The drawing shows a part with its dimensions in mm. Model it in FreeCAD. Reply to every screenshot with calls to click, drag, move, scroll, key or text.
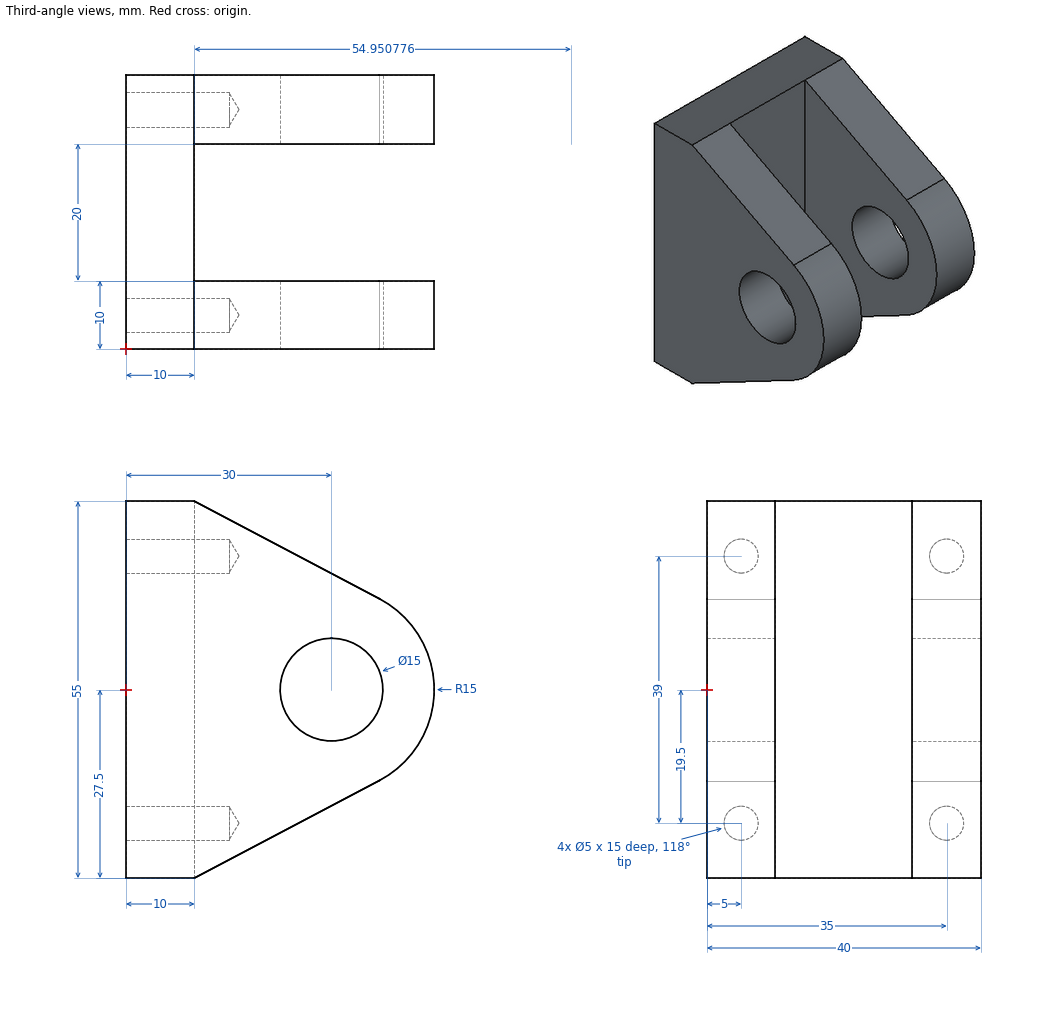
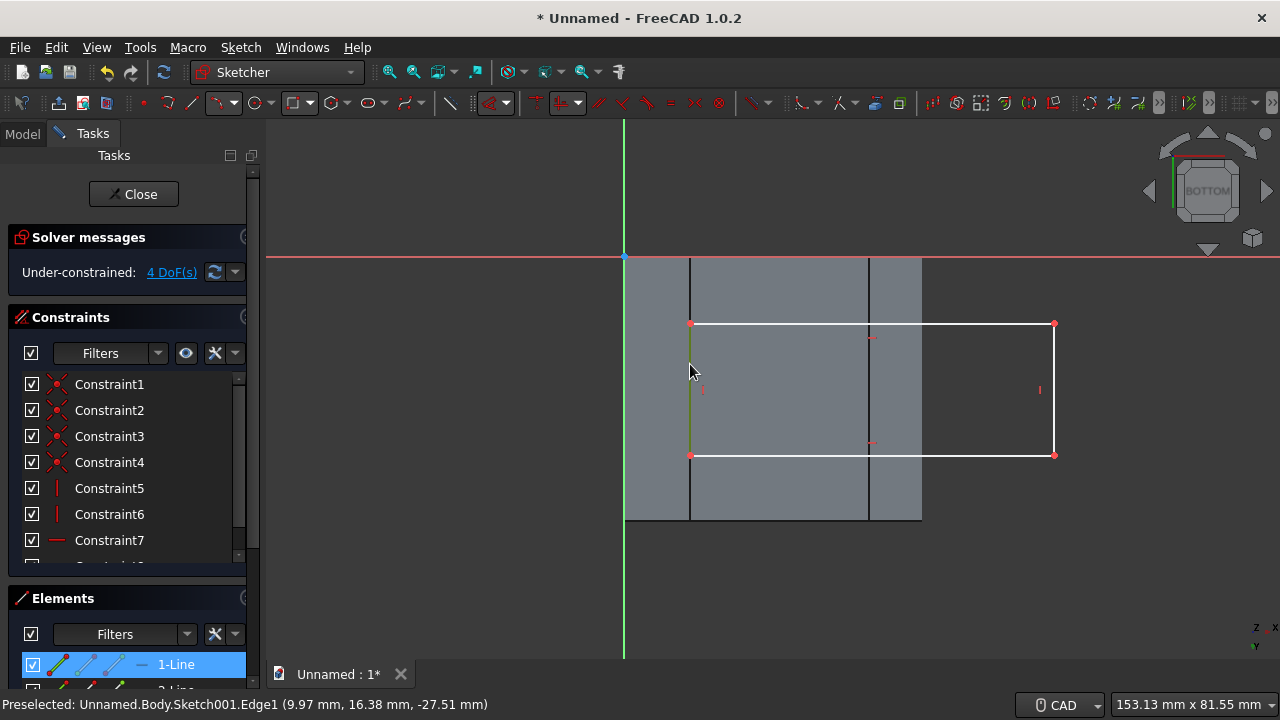
key(i)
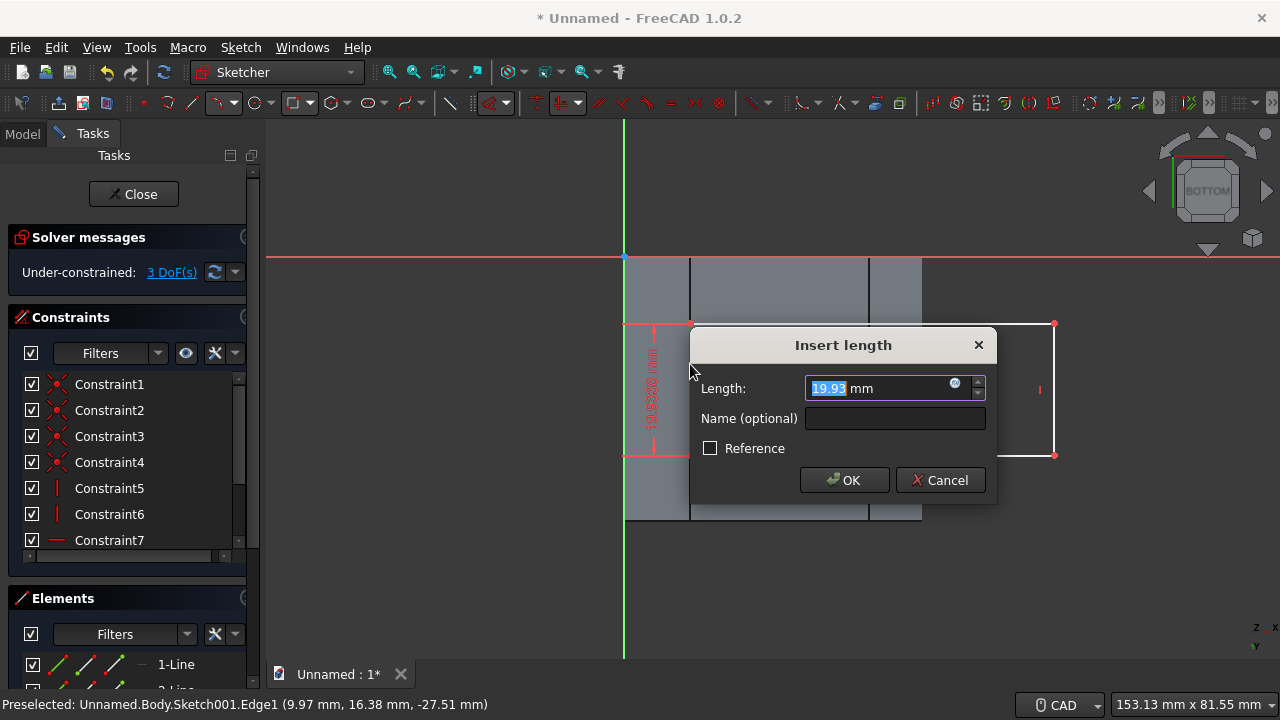
text(20)
key(Return)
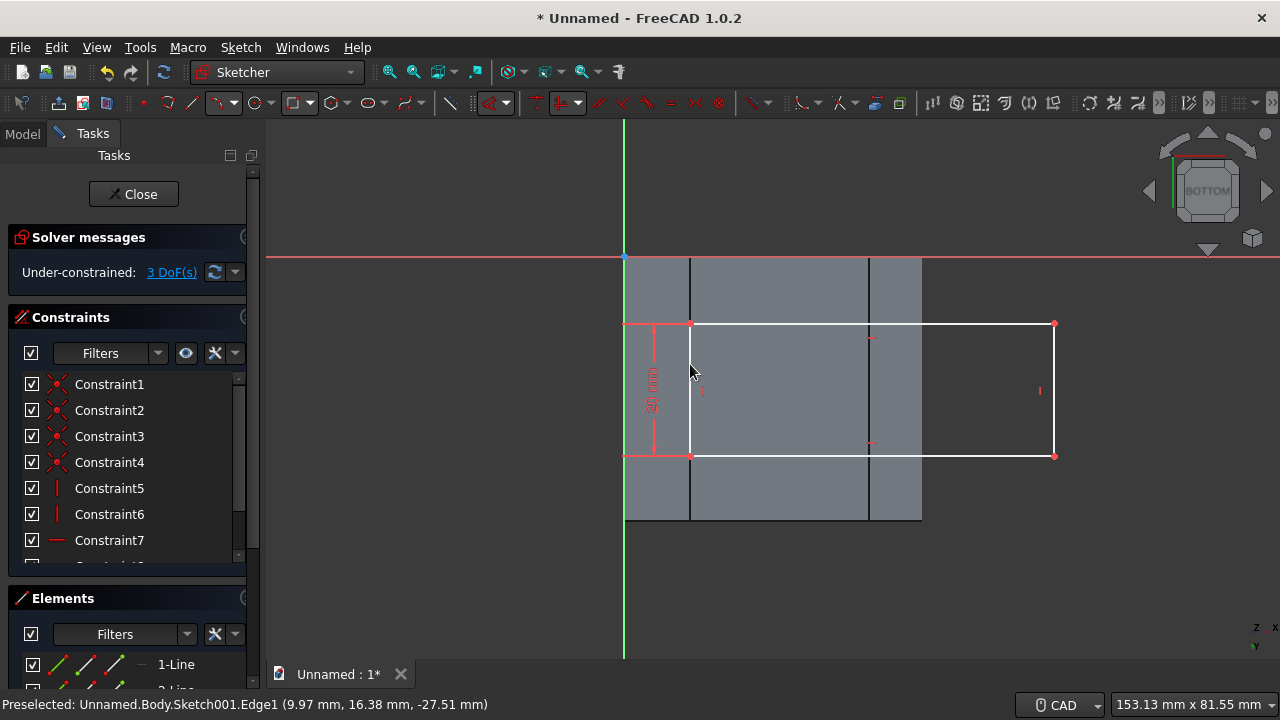
click(690, 324)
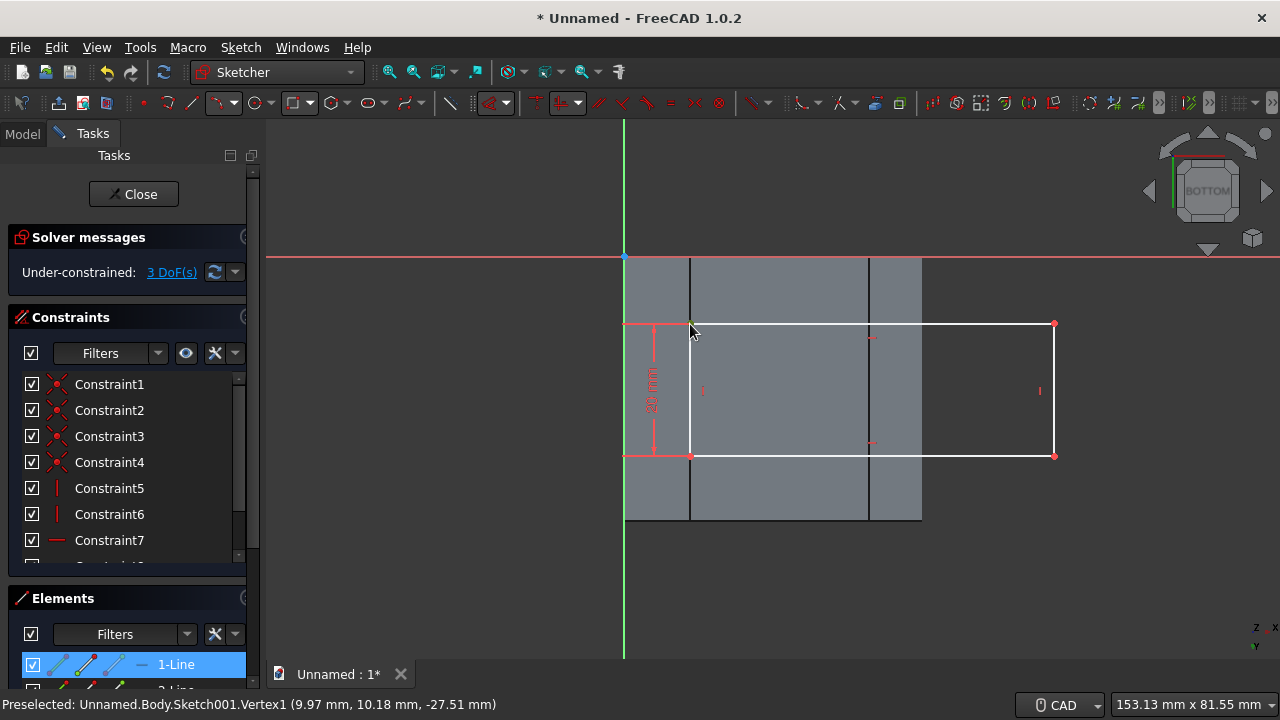
key(l)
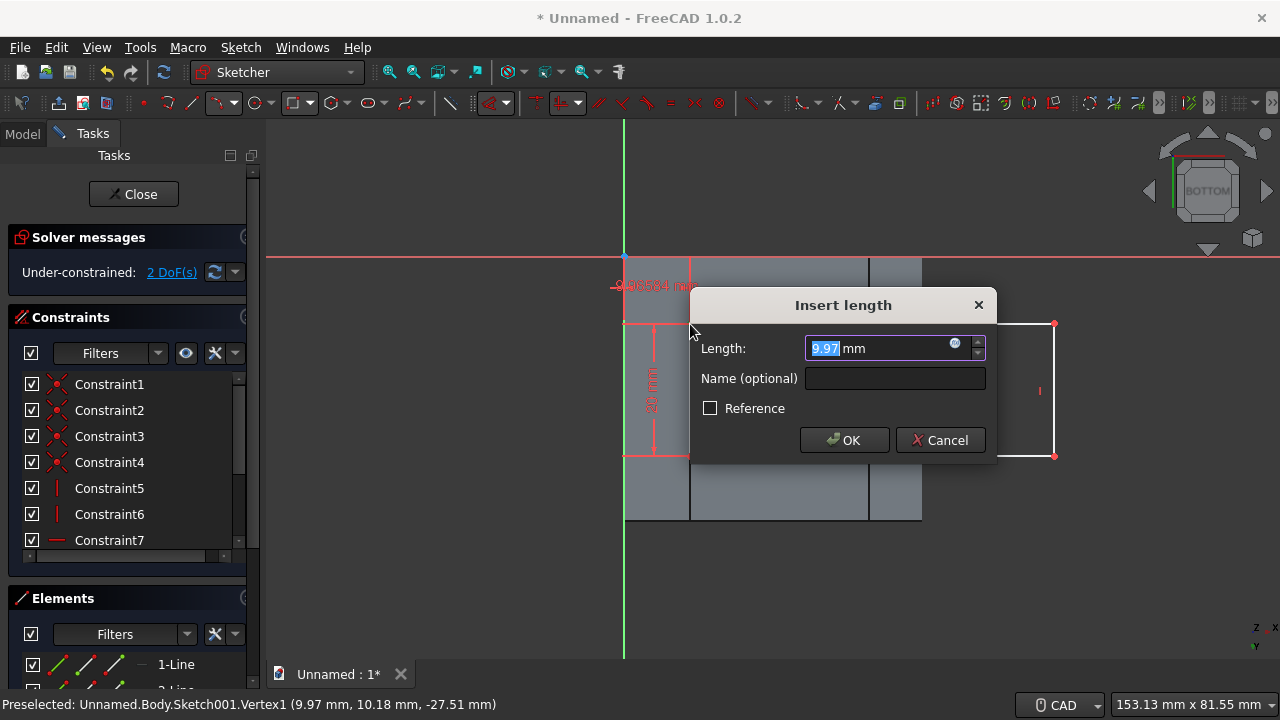
text(10)
key(Return)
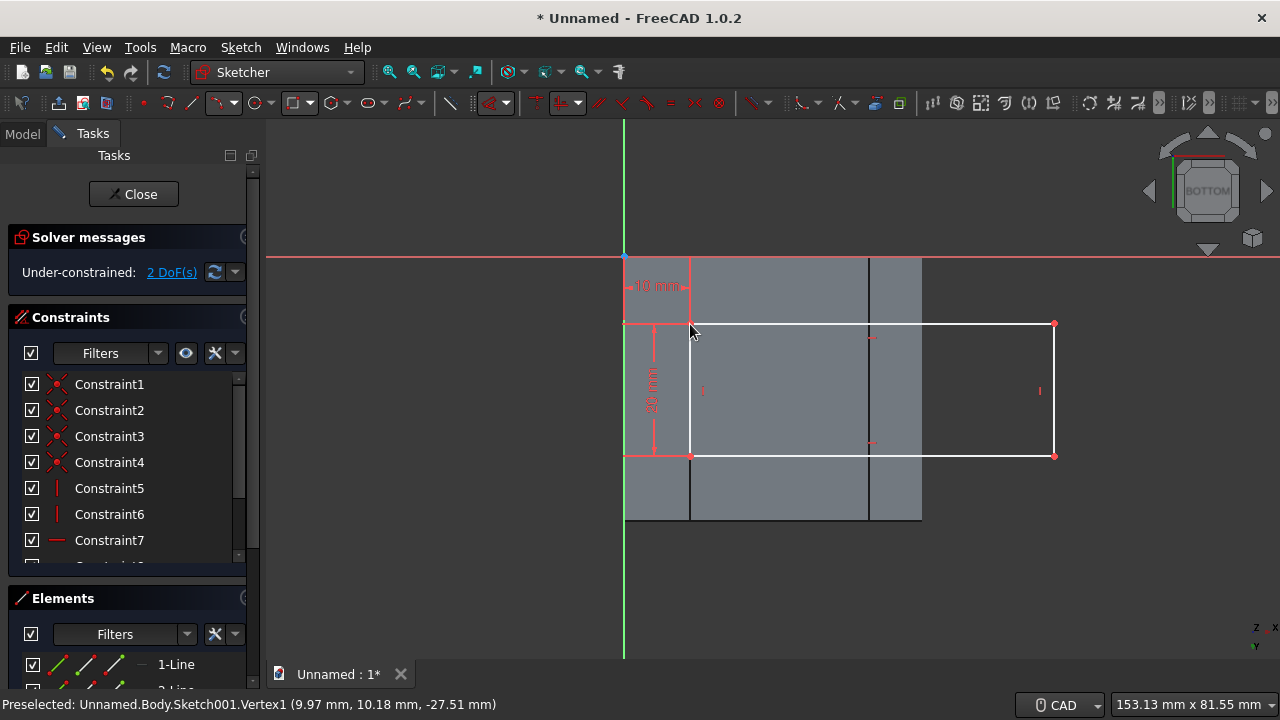
click(690, 324)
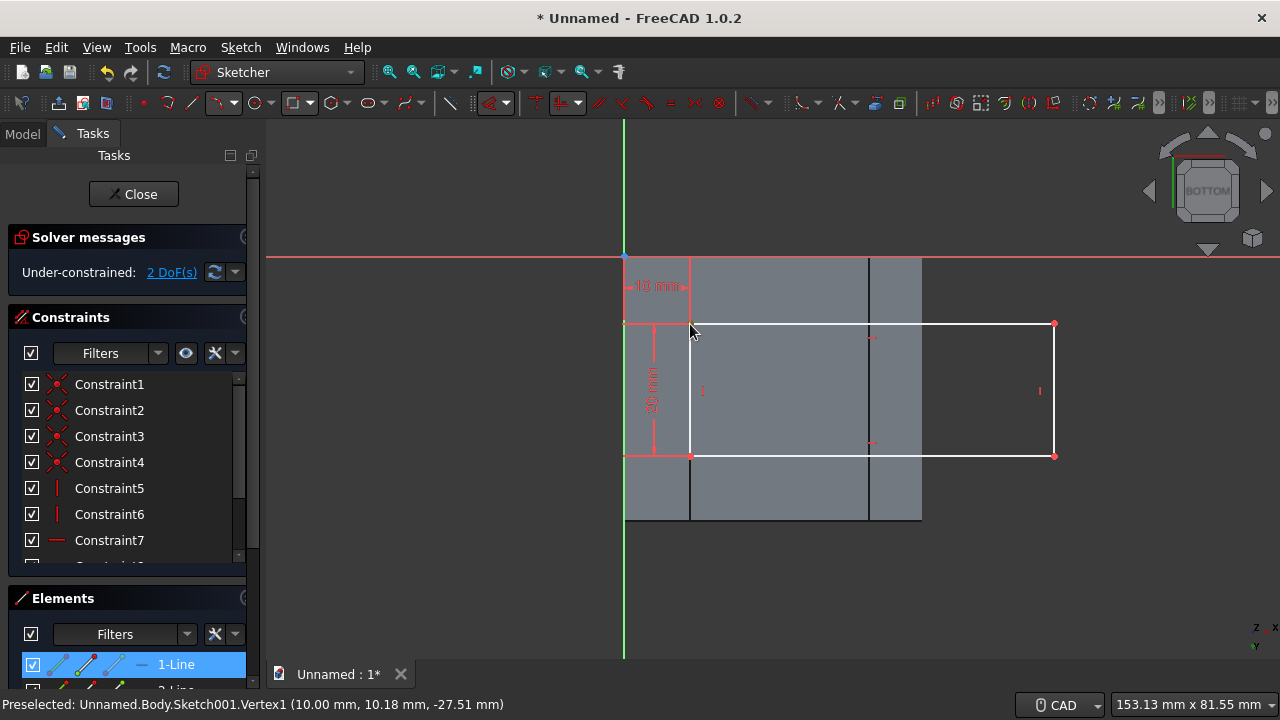
key(i)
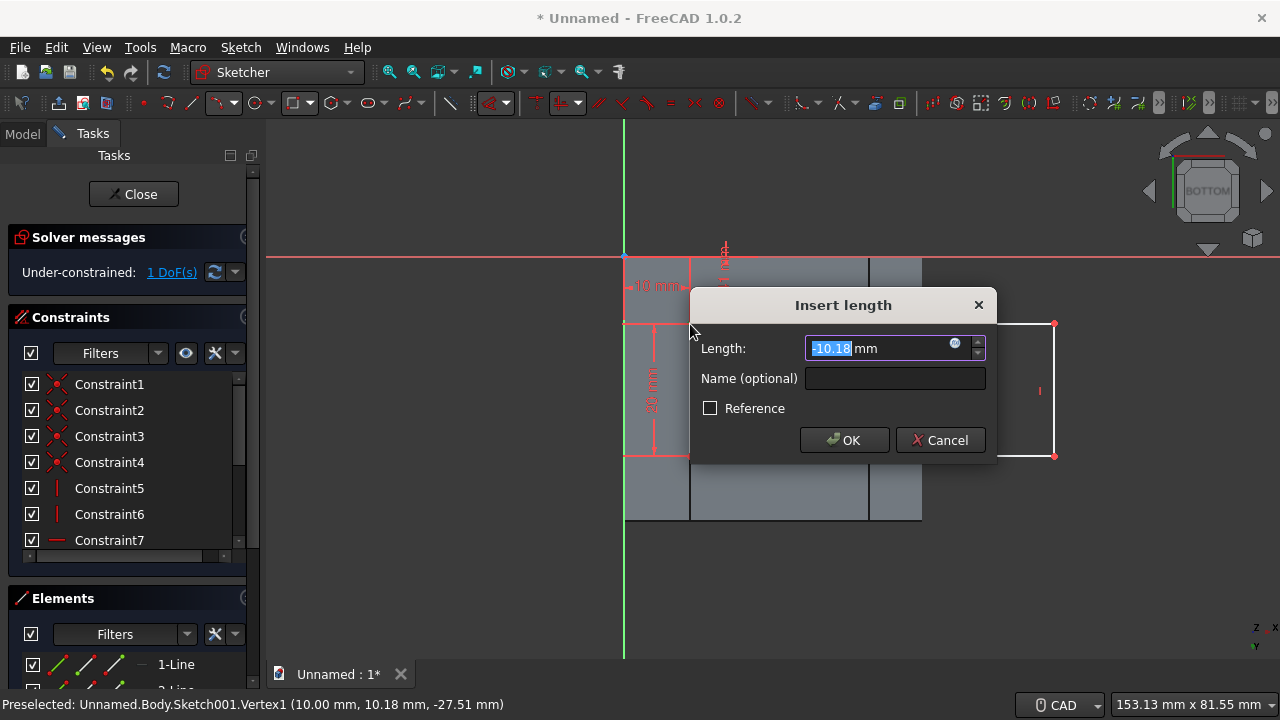
text(-10)
key(Return)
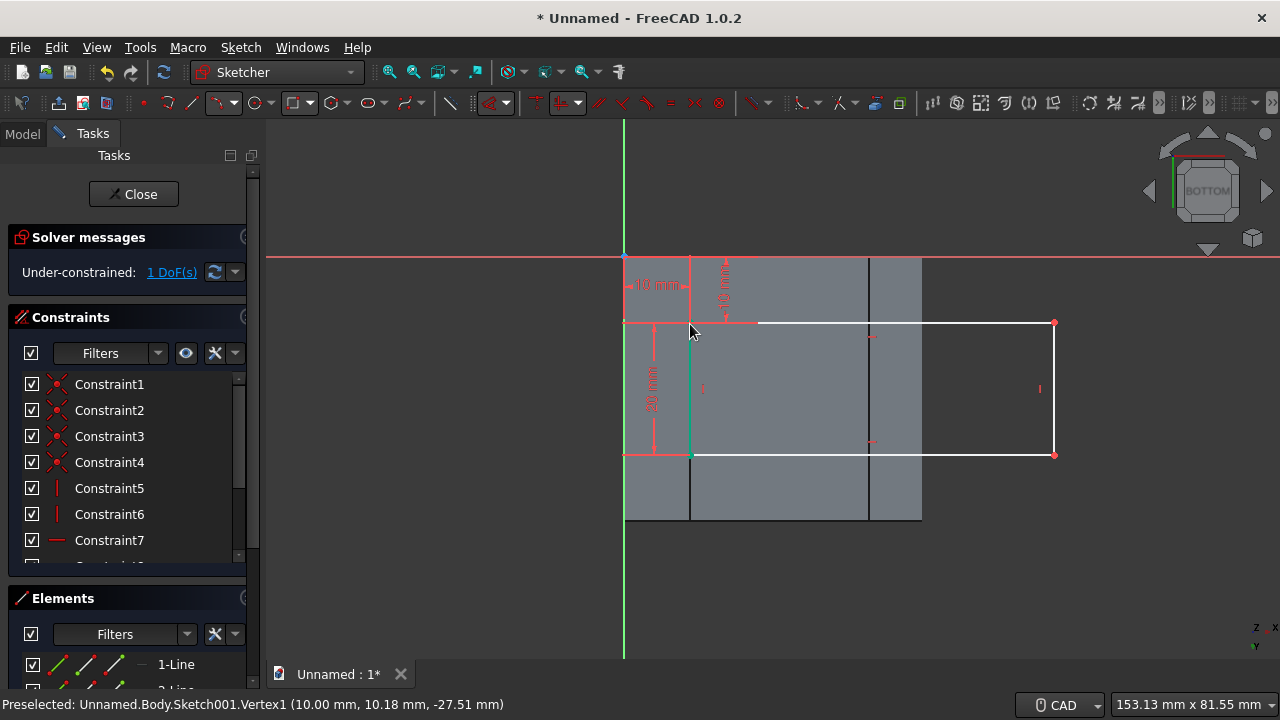
click(799, 455)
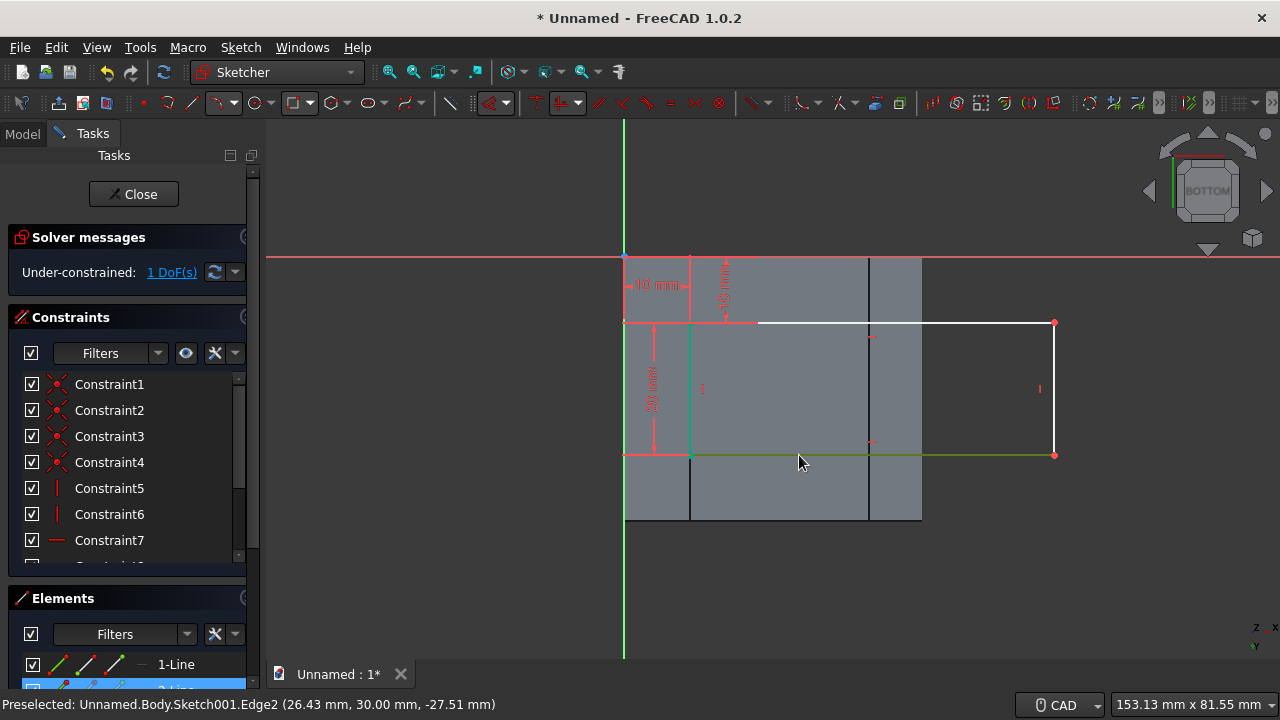
key(l)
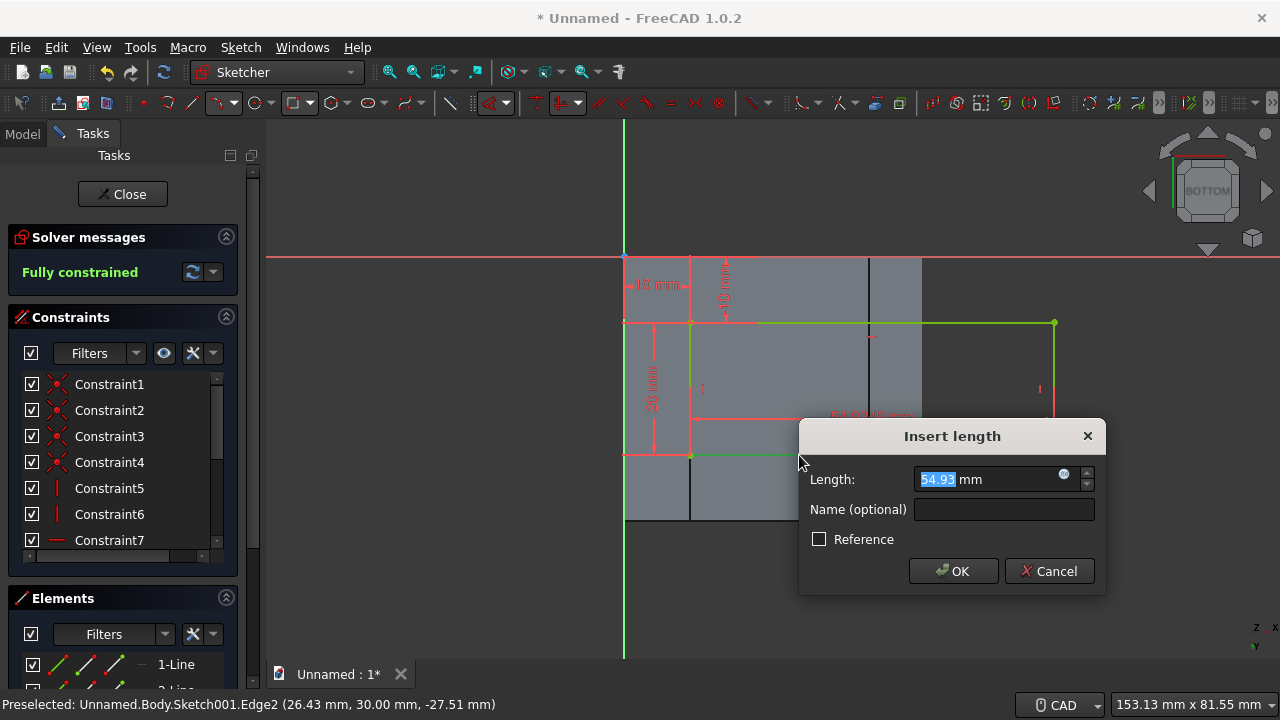
text(54.950776)
key(Return)